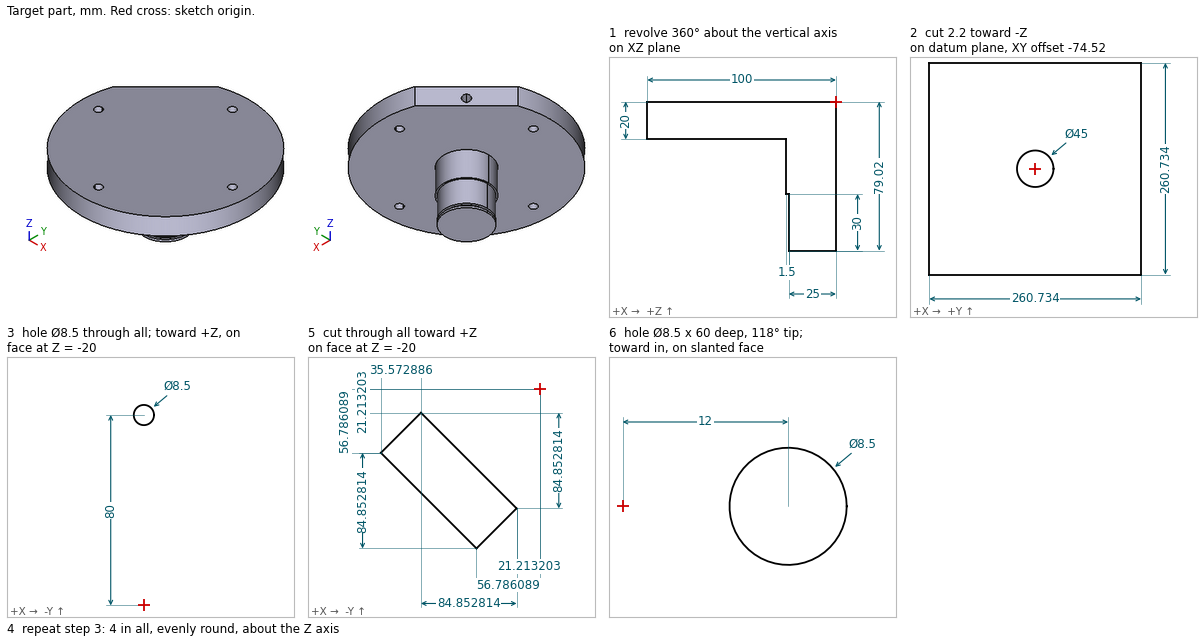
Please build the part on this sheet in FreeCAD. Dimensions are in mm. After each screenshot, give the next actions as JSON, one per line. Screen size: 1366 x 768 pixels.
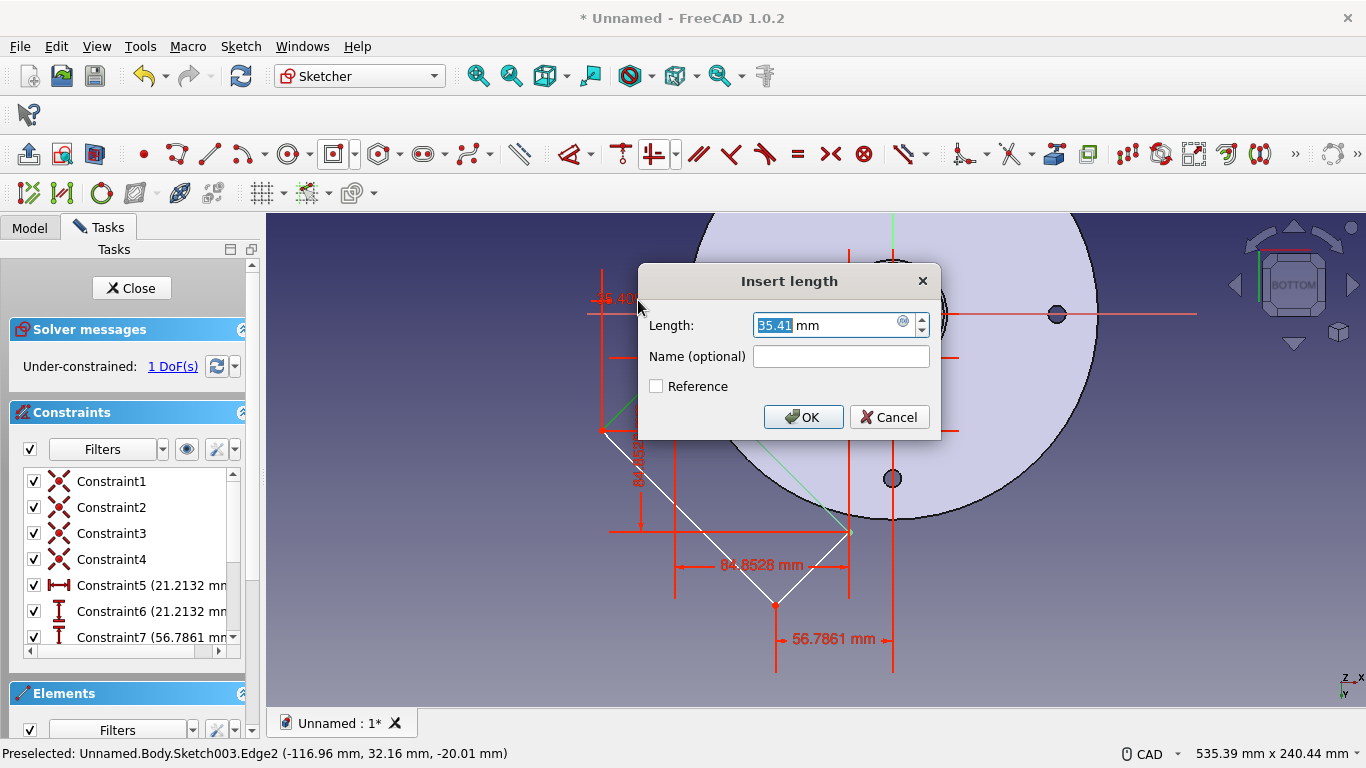
{"action": "type", "text": "35.572886"}
{"action": "key", "text": "Return"}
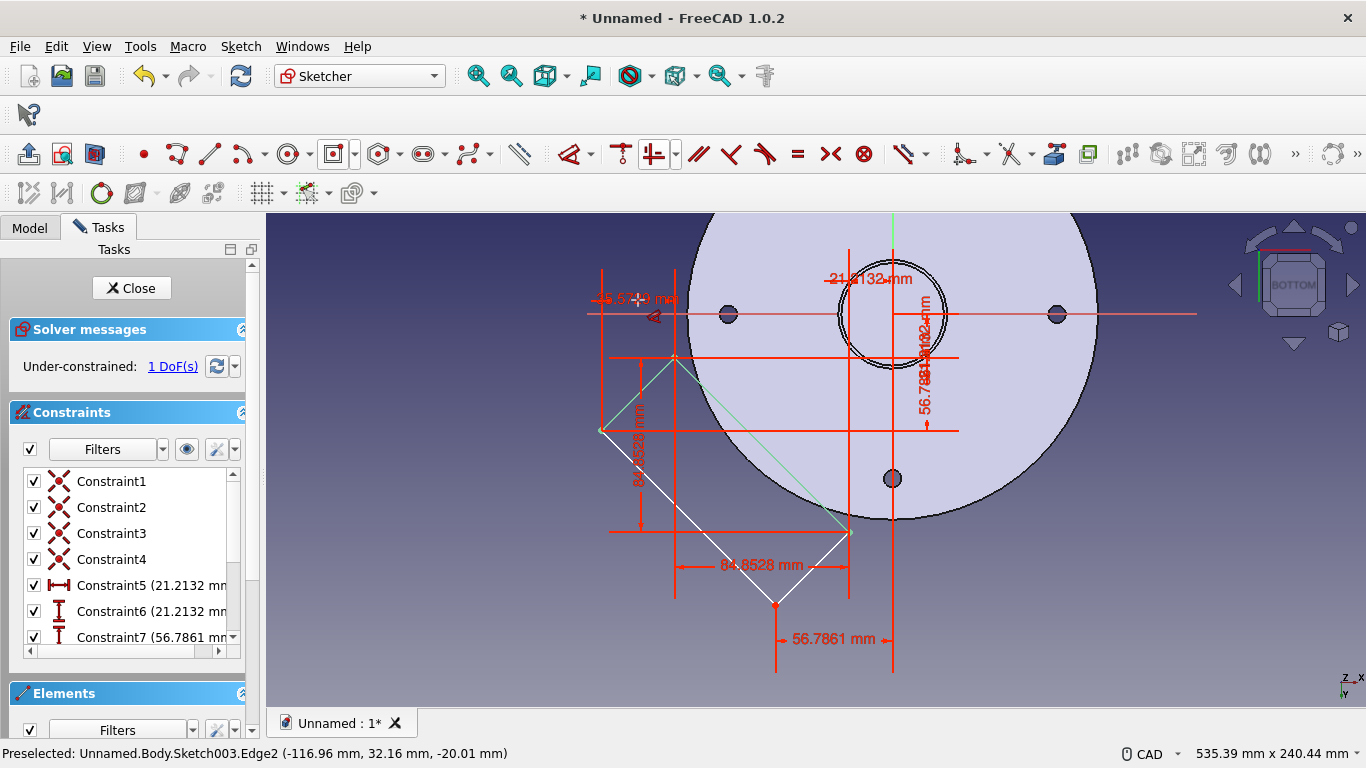
{"action": "left_click", "coordinate": [654, 483]}
{"action": "left_click", "coordinate": [568, 518]}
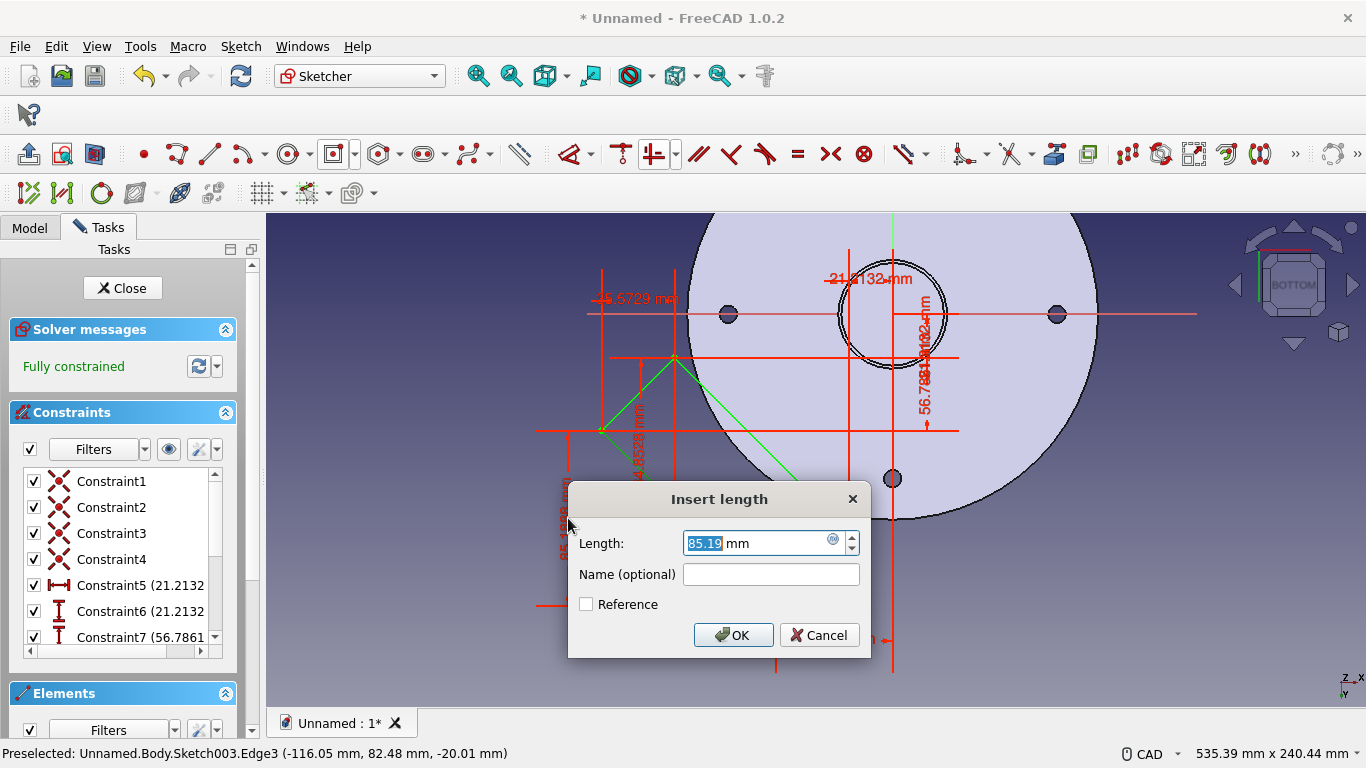
{"action": "type", "text": "84.852814"}
{"action": "key", "text": "Return"}
{"action": "key", "text": "Escape"}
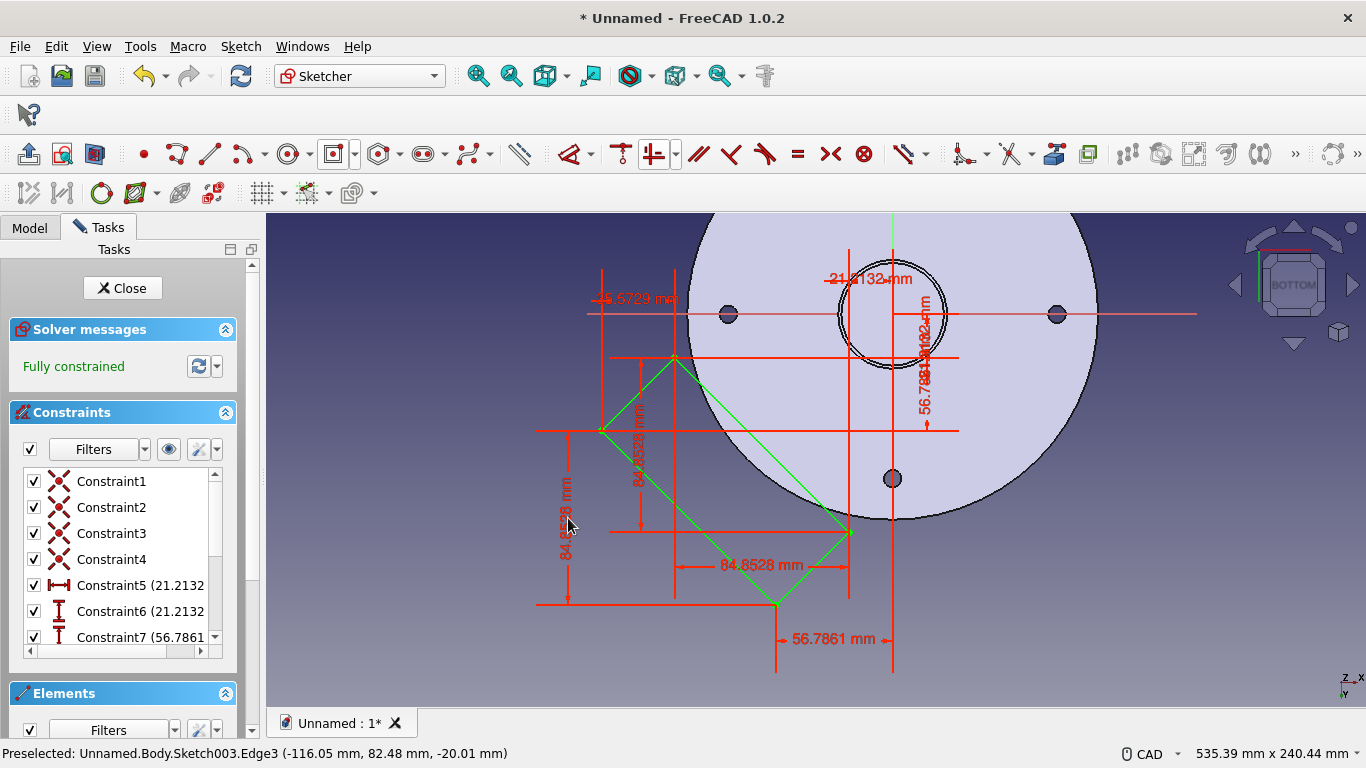
{"action": "left_click", "coordinate": [123, 288]}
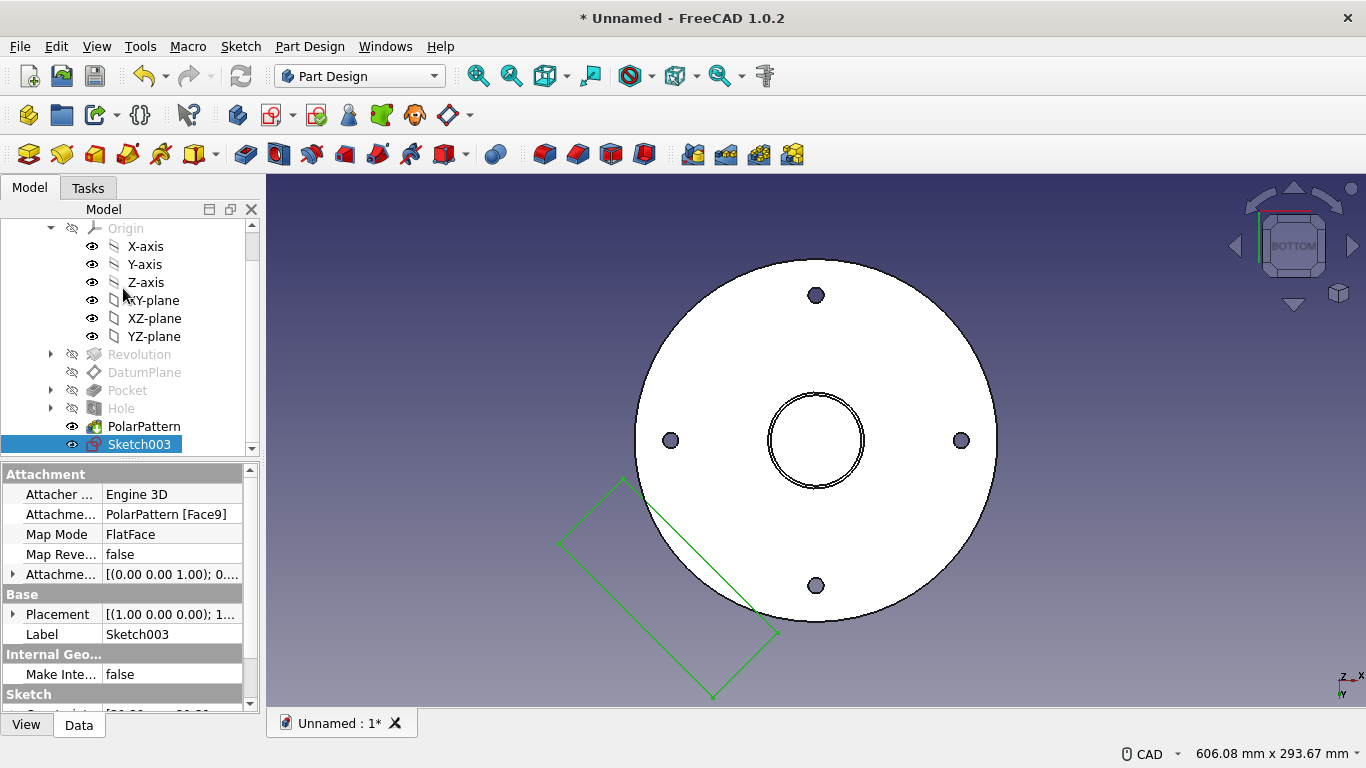
{"action": "left_click", "coordinate": [246, 154]}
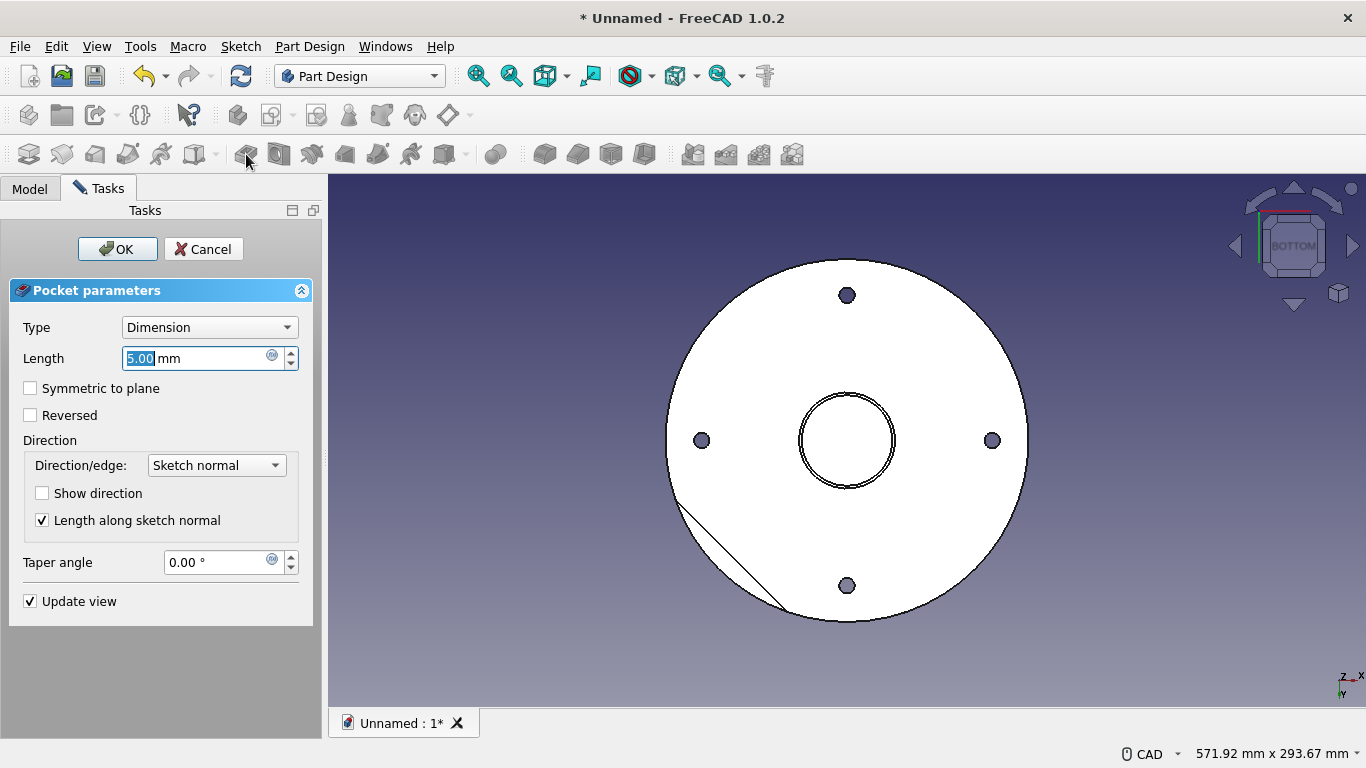
{"action": "left_click", "coordinate": [210, 328]}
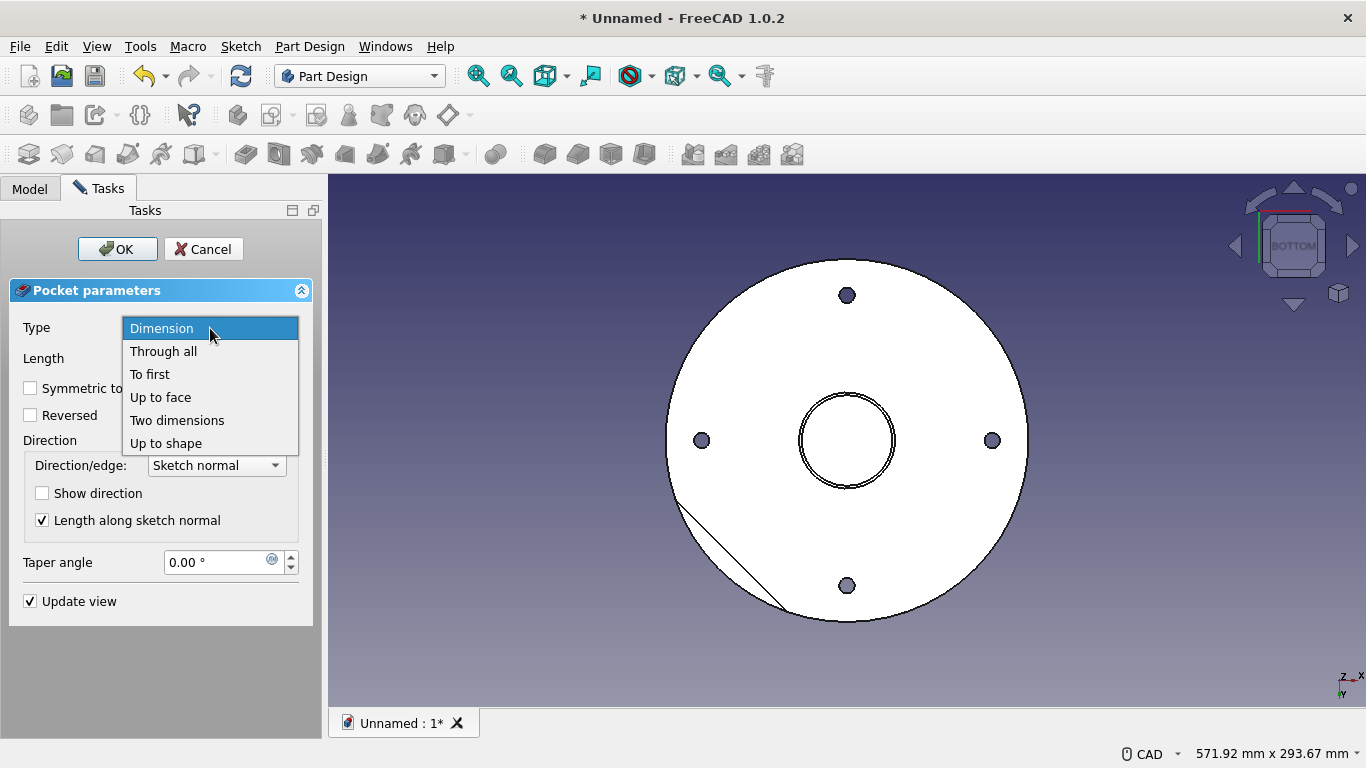
{"action": "left_click", "coordinate": [208, 352]}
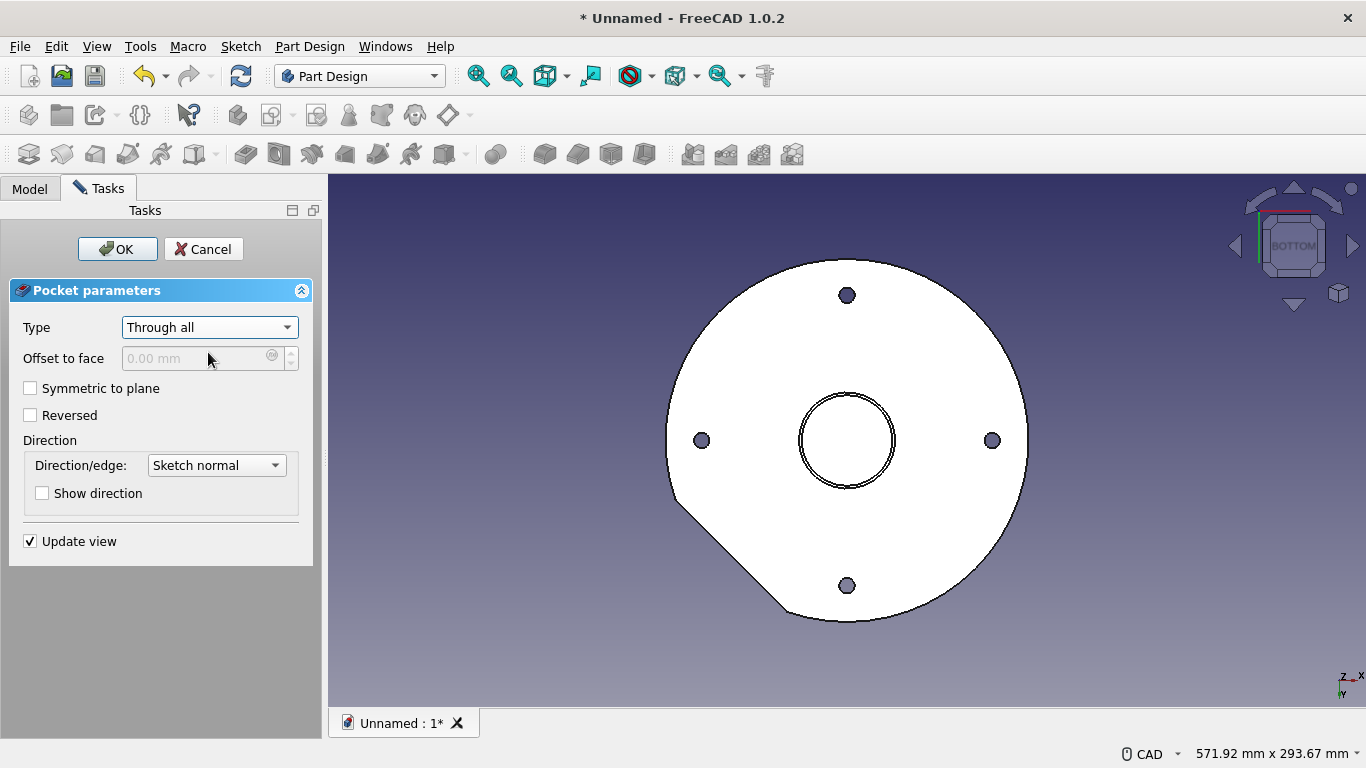
{"action": "left_click", "coordinate": [118, 249]}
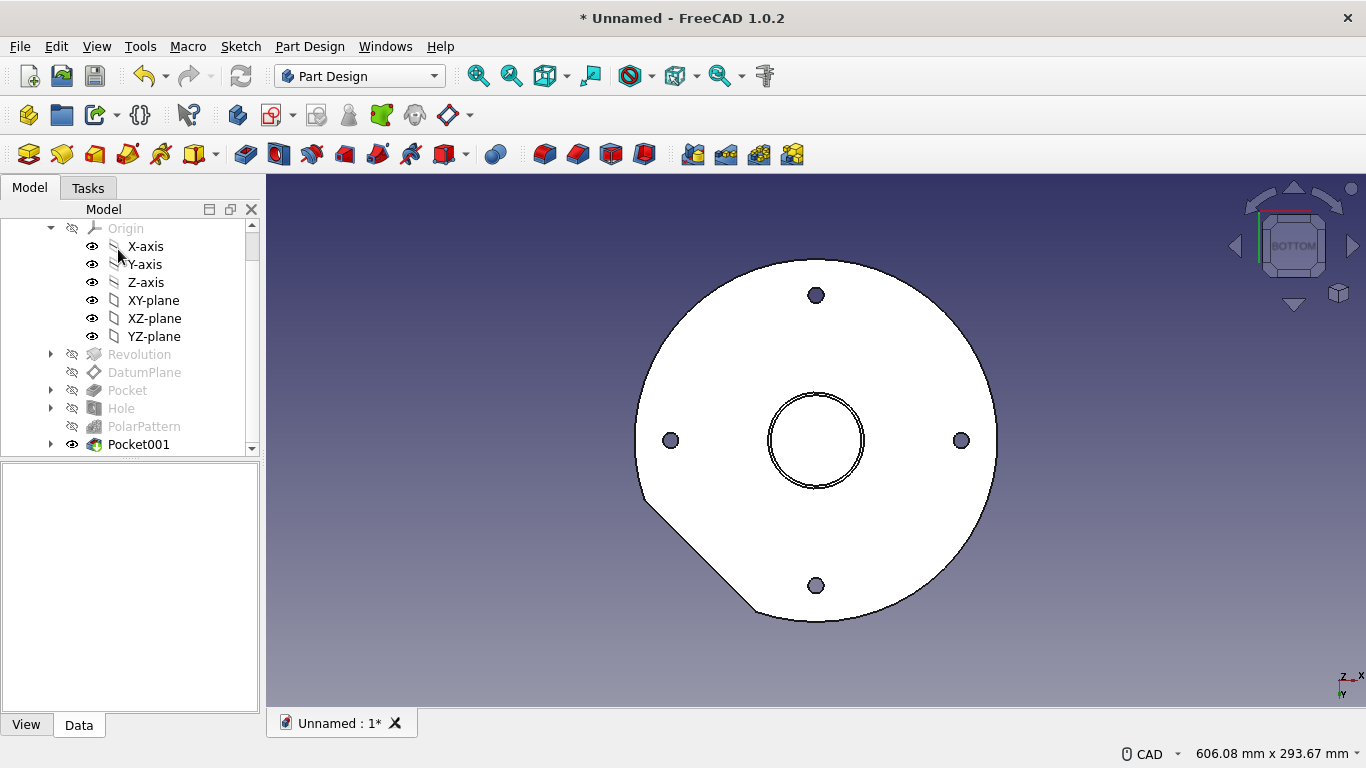
{"action": "key", "text": "4"}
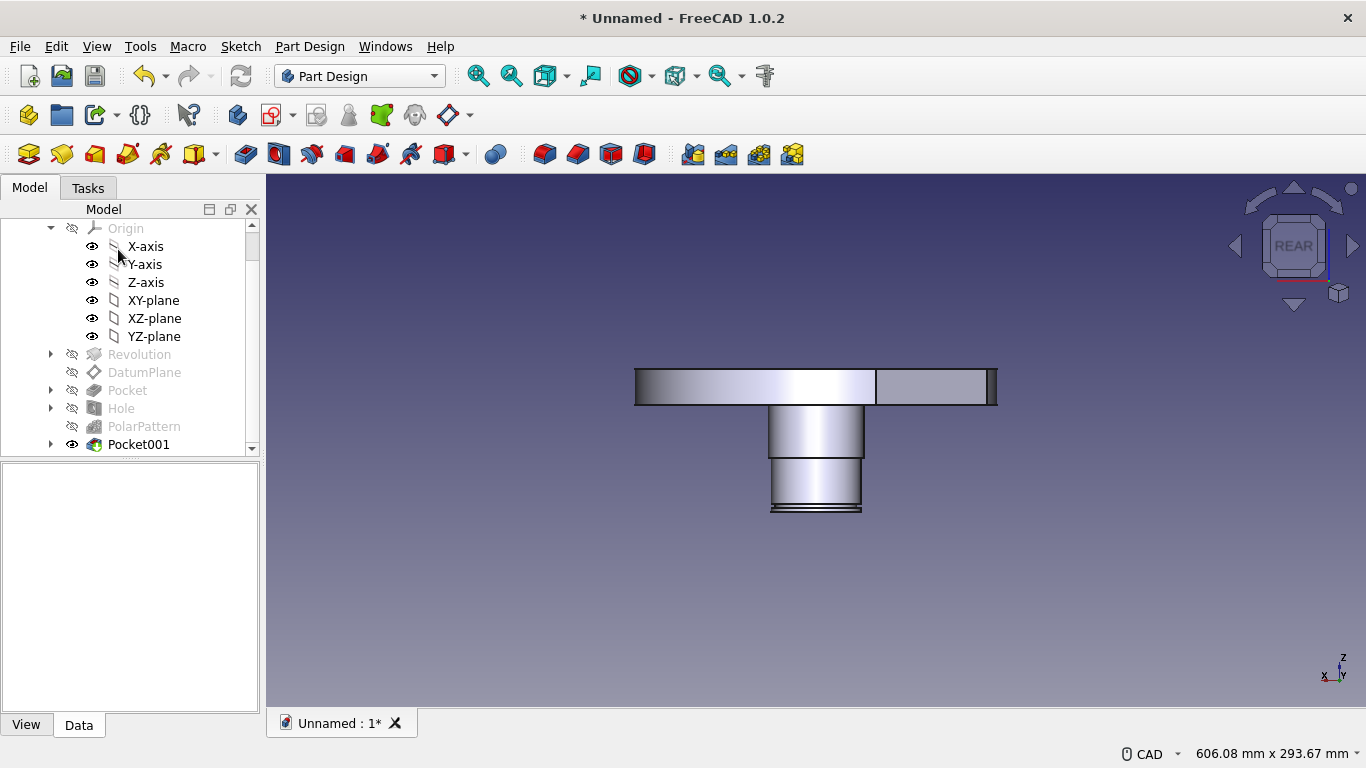
{"action": "left_click", "coordinate": [479, 76]}